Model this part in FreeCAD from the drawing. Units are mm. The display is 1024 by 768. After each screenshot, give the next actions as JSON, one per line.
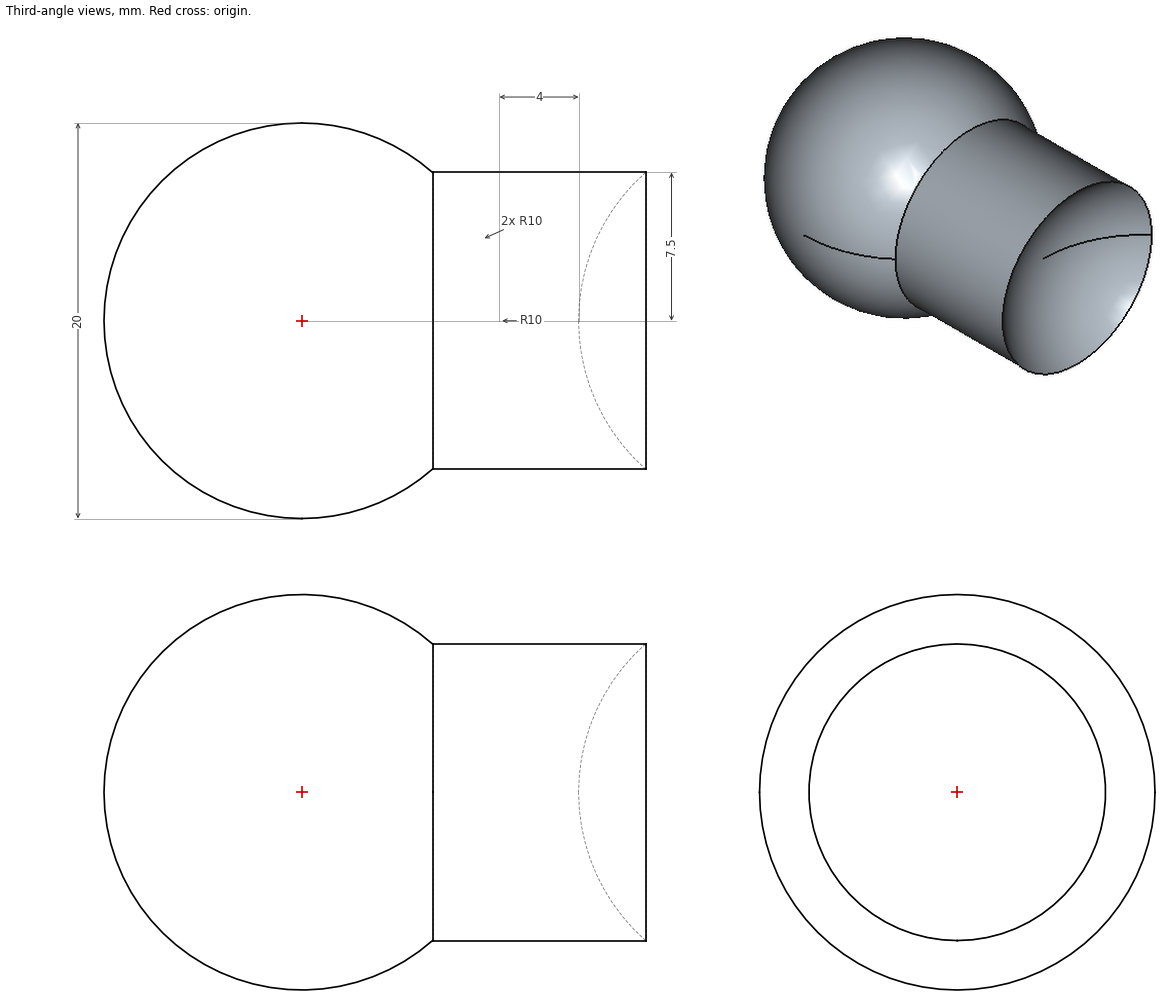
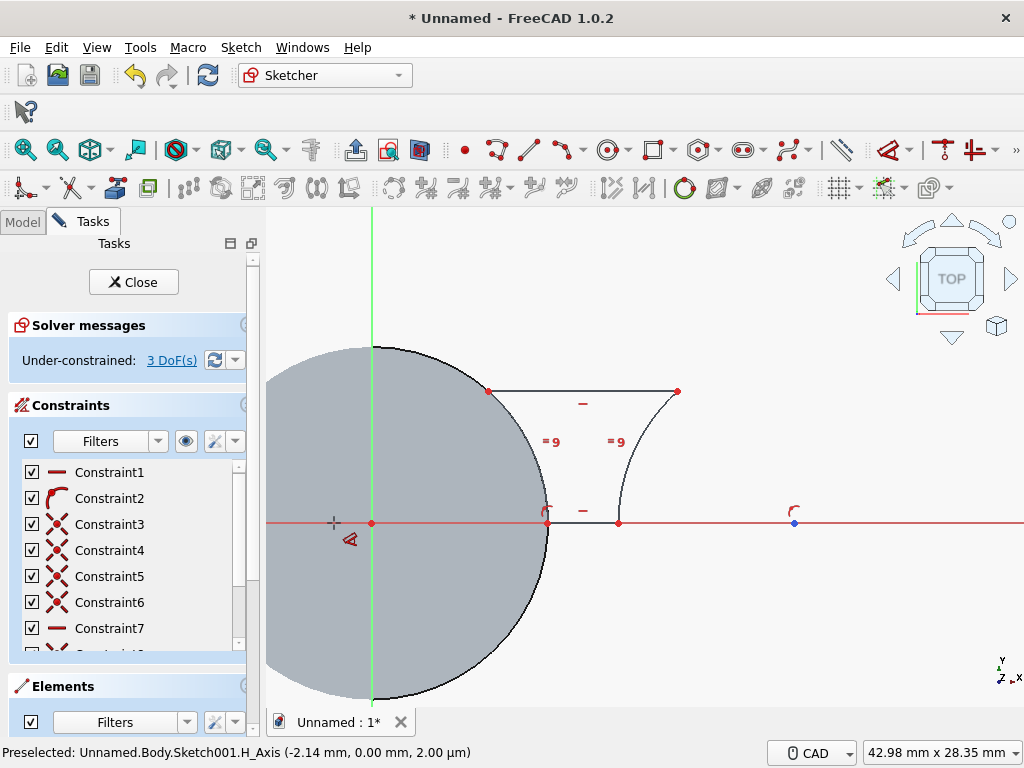
{"action": "left_click", "coordinate": [542, 479]}
{"action": "left_click", "coordinate": [573, 471]}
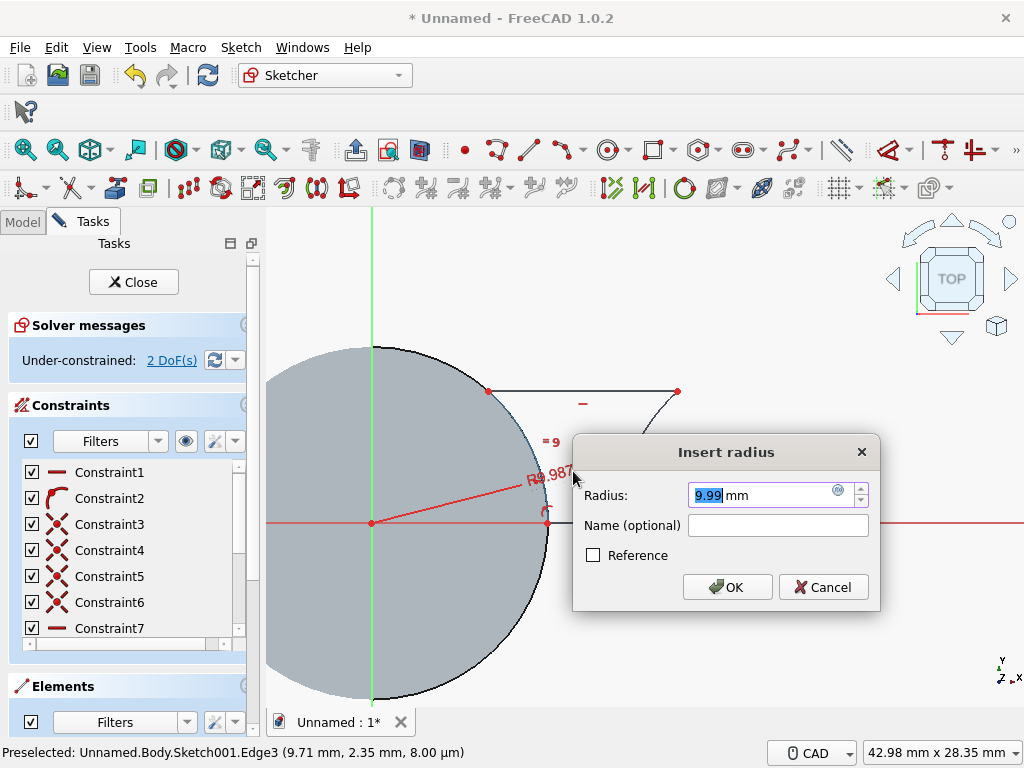
{"action": "type", "text": "10"}
{"action": "key", "text": "Return"}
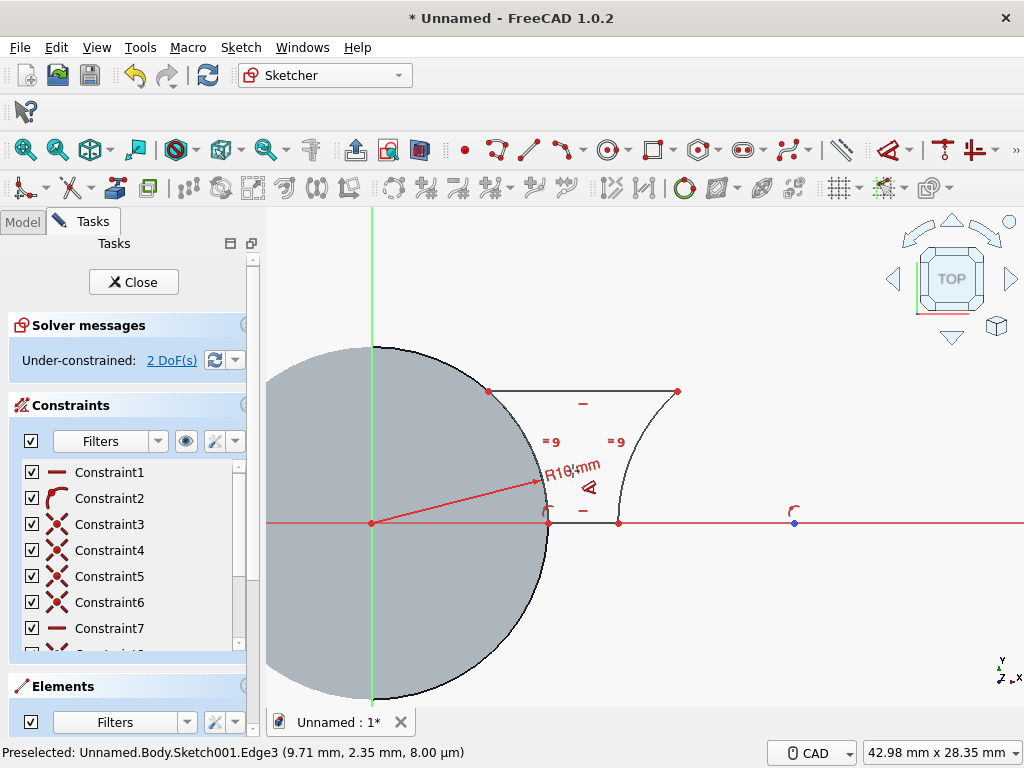
{"action": "left_click", "coordinate": [569, 523]}
{"action": "left_click", "coordinate": [583, 557]}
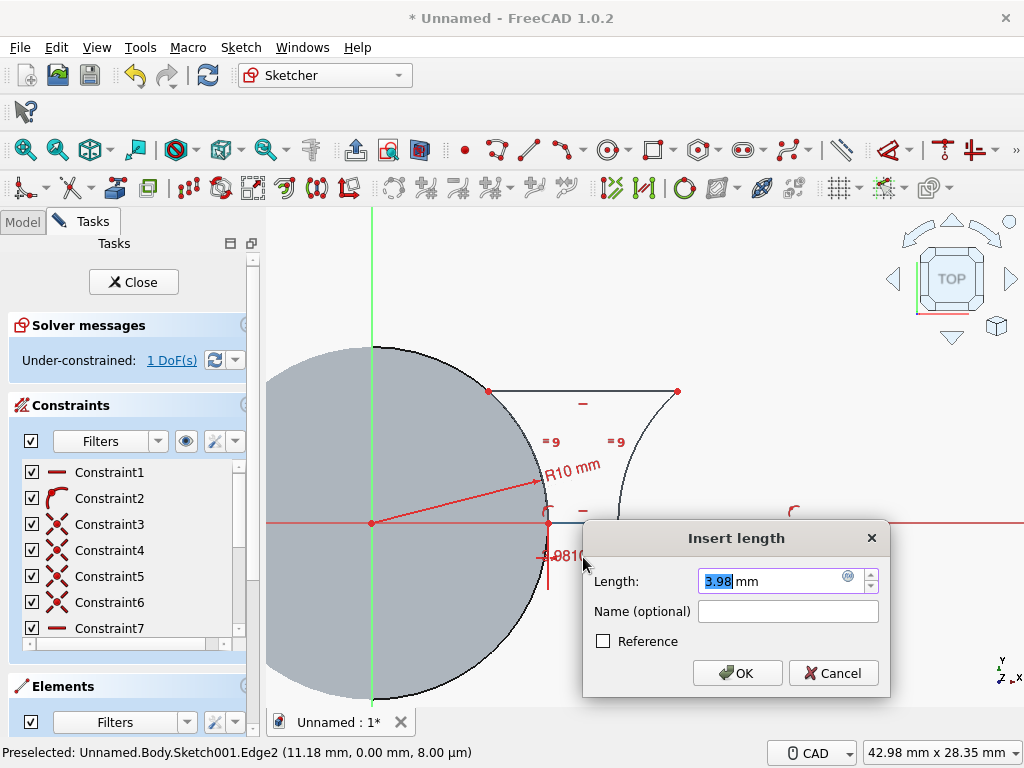
{"action": "type", "text": "4"}
{"action": "key", "text": "Return"}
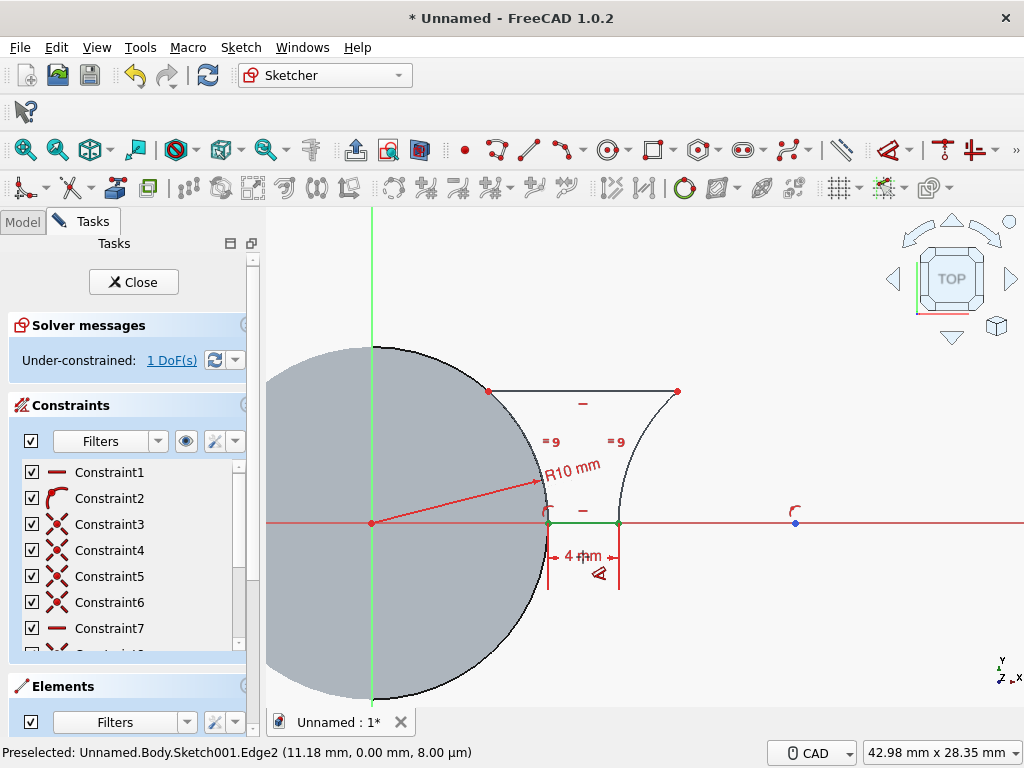
{"action": "left_click", "coordinate": [678, 391]}
{"action": "left_click", "coordinate": [338, 457]}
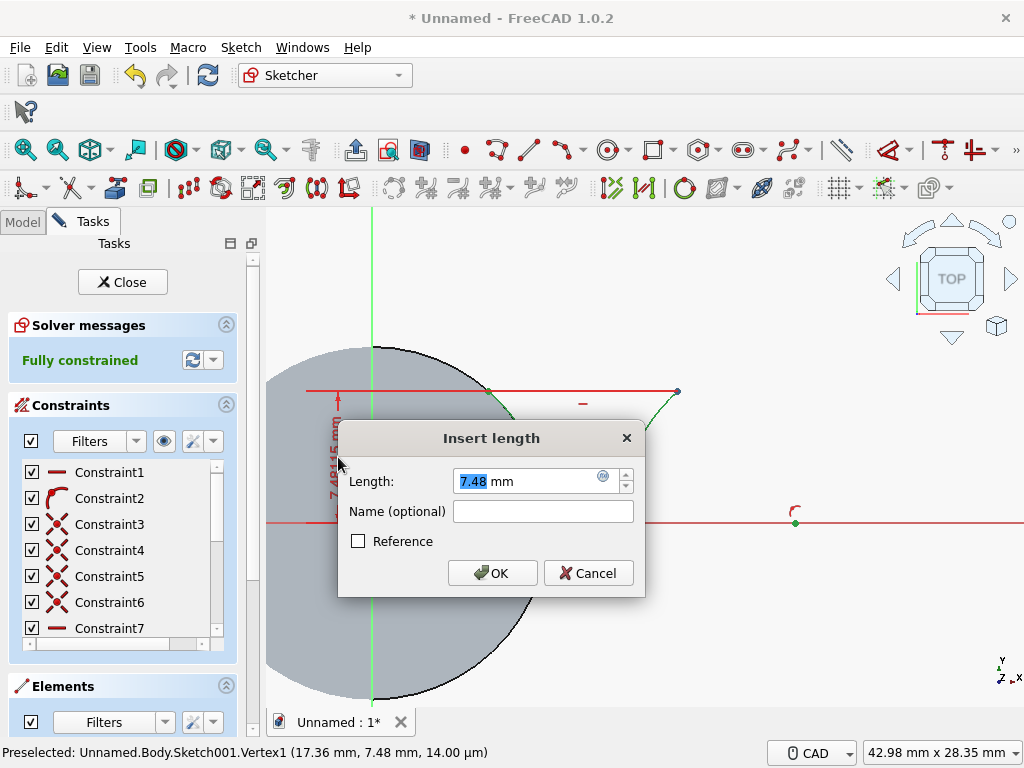
{"action": "type", "text": "7.5"}
{"action": "key", "text": "Return"}
{"action": "key", "text": "Escape"}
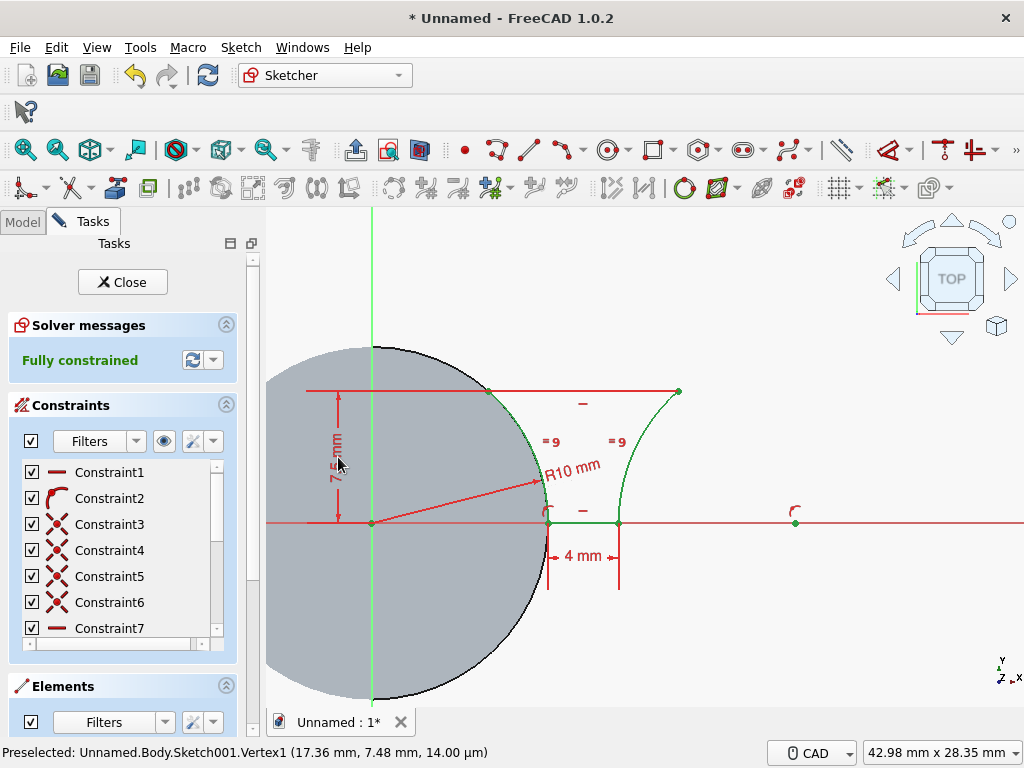
{"action": "left_click", "coordinate": [123, 282]}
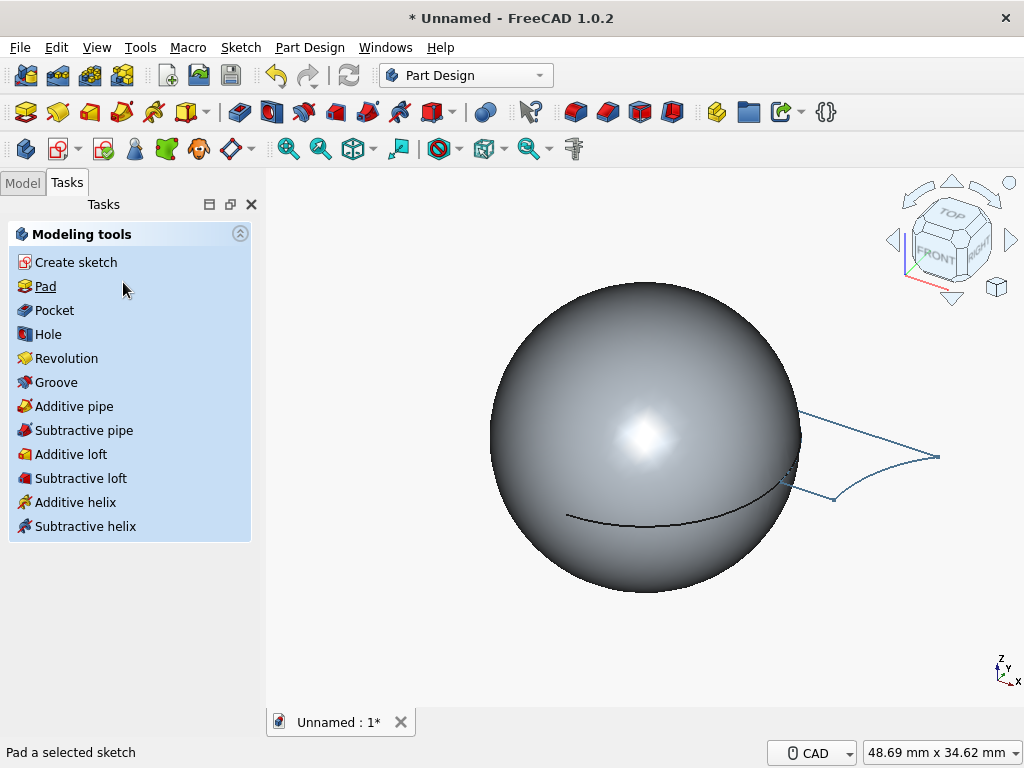
{"action": "left_click", "coordinate": [58, 112]}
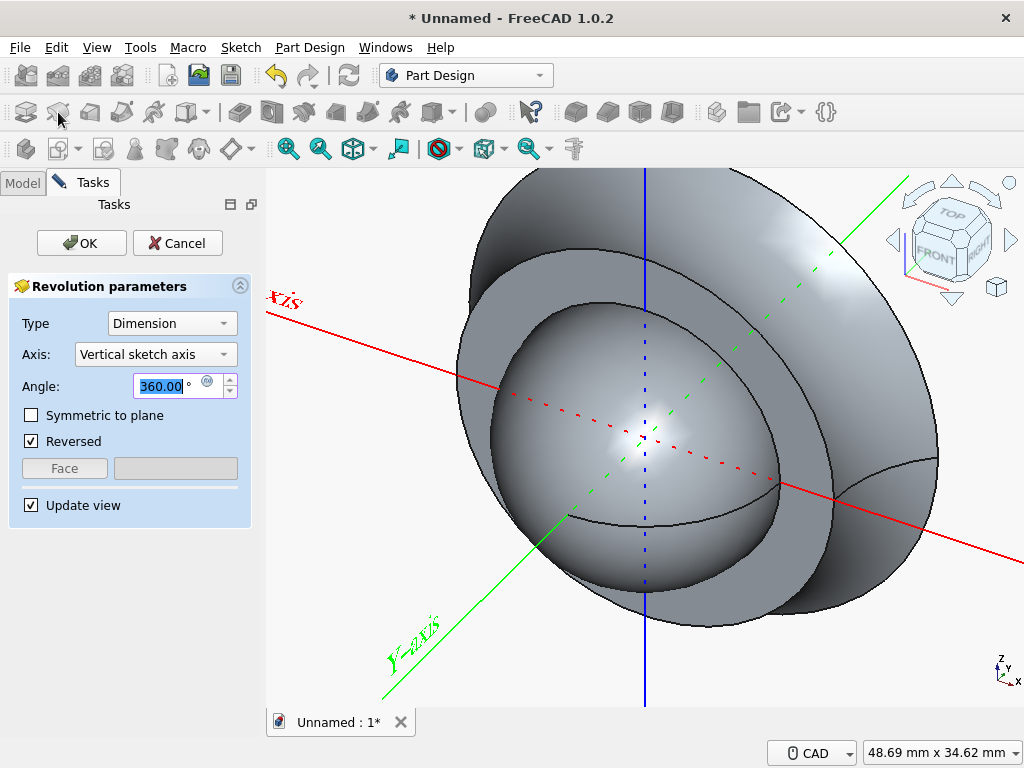
{"action": "left_click", "coordinate": [156, 354]}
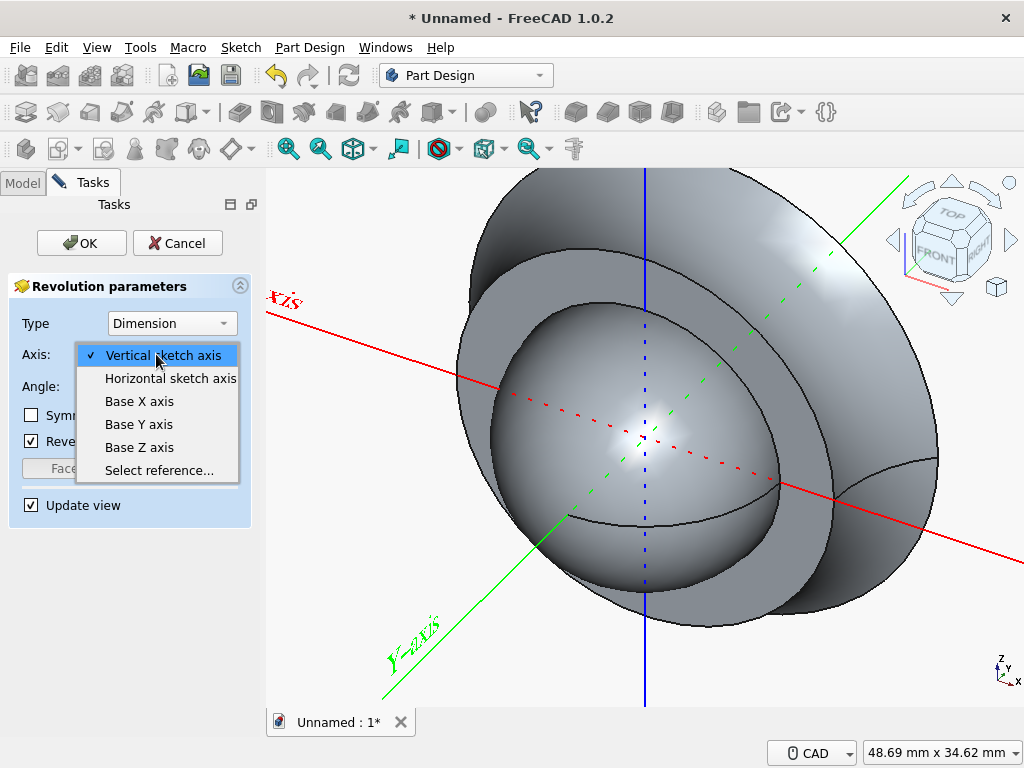
{"action": "left_click", "coordinate": [156, 378]}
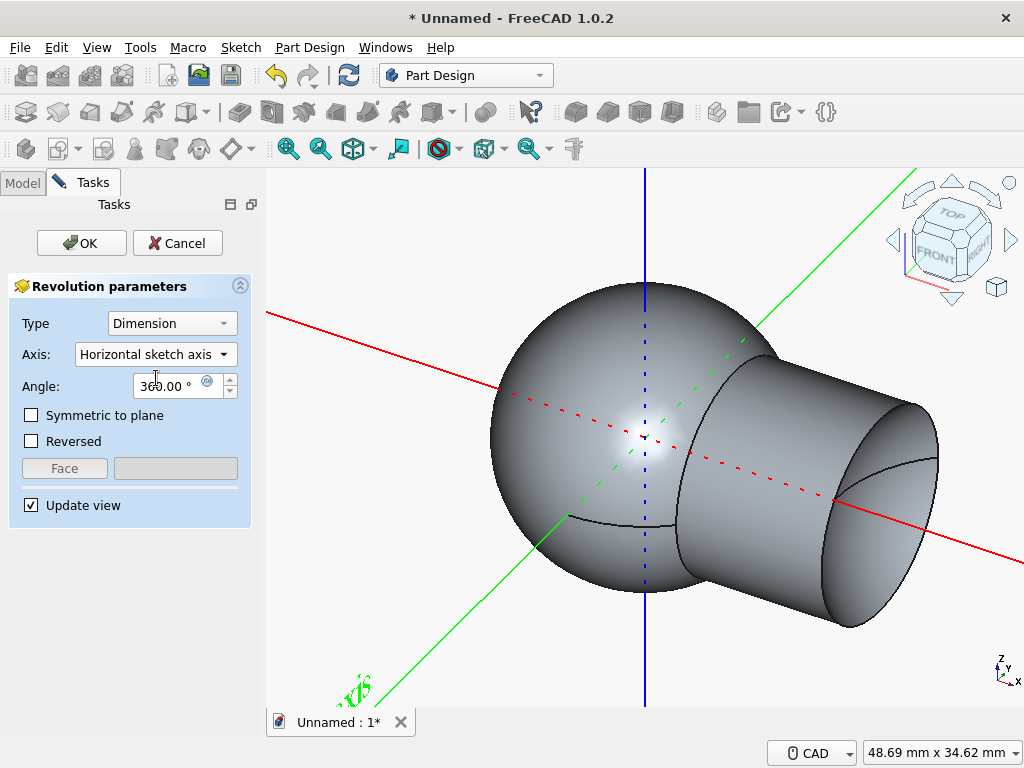
{"action": "left_click", "coordinate": [82, 243]}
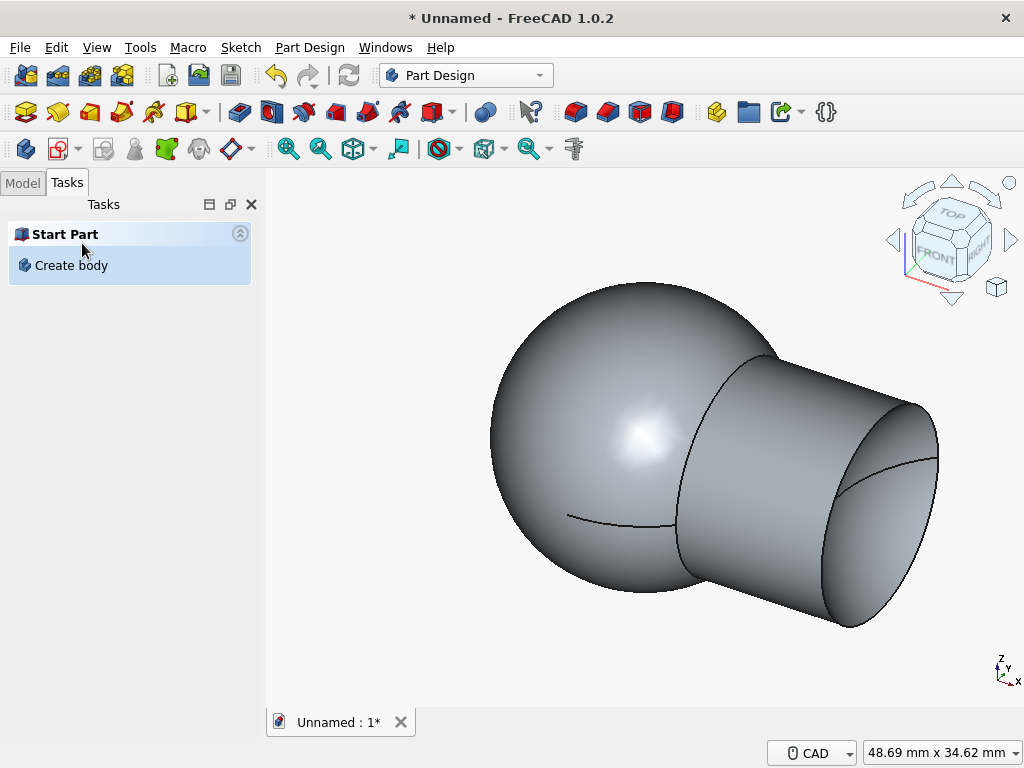
{"action": "key", "text": "0"}